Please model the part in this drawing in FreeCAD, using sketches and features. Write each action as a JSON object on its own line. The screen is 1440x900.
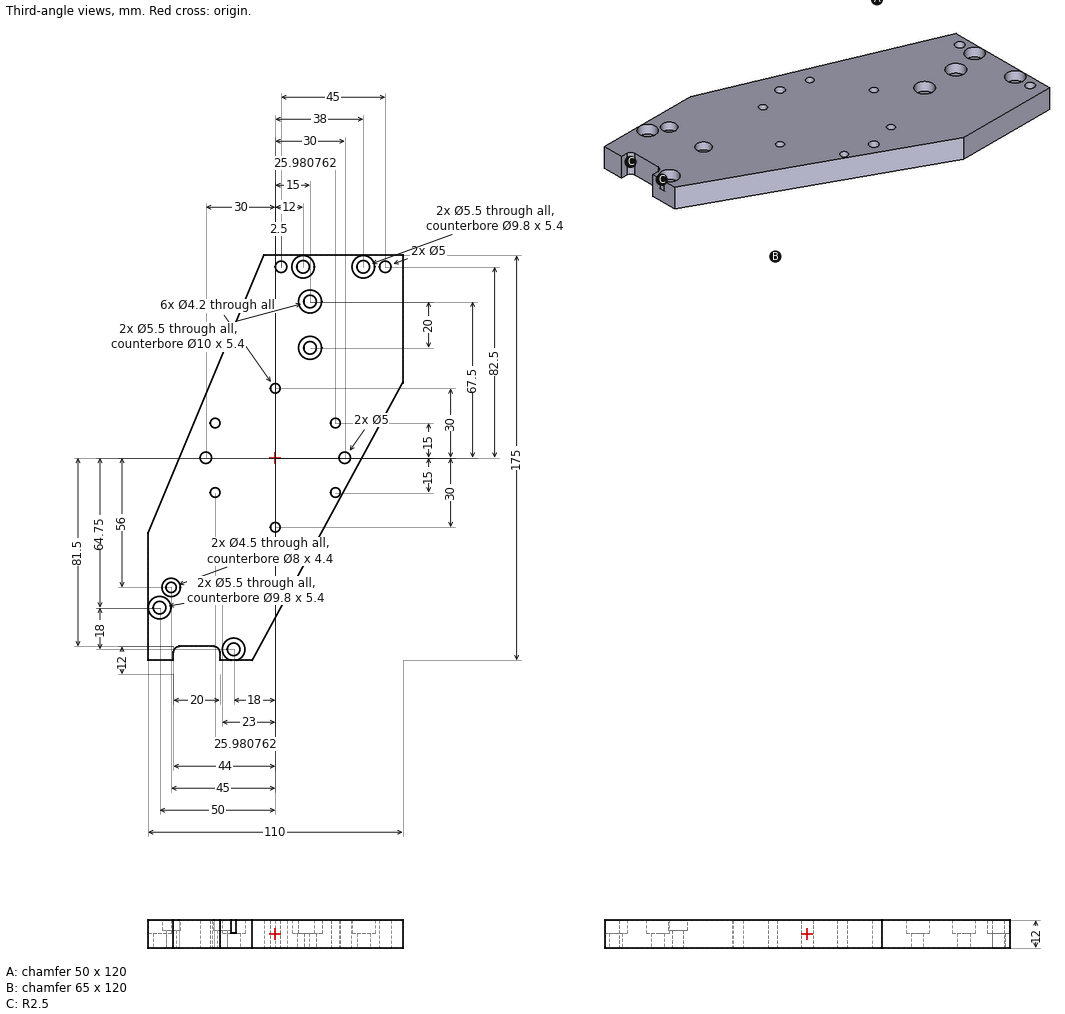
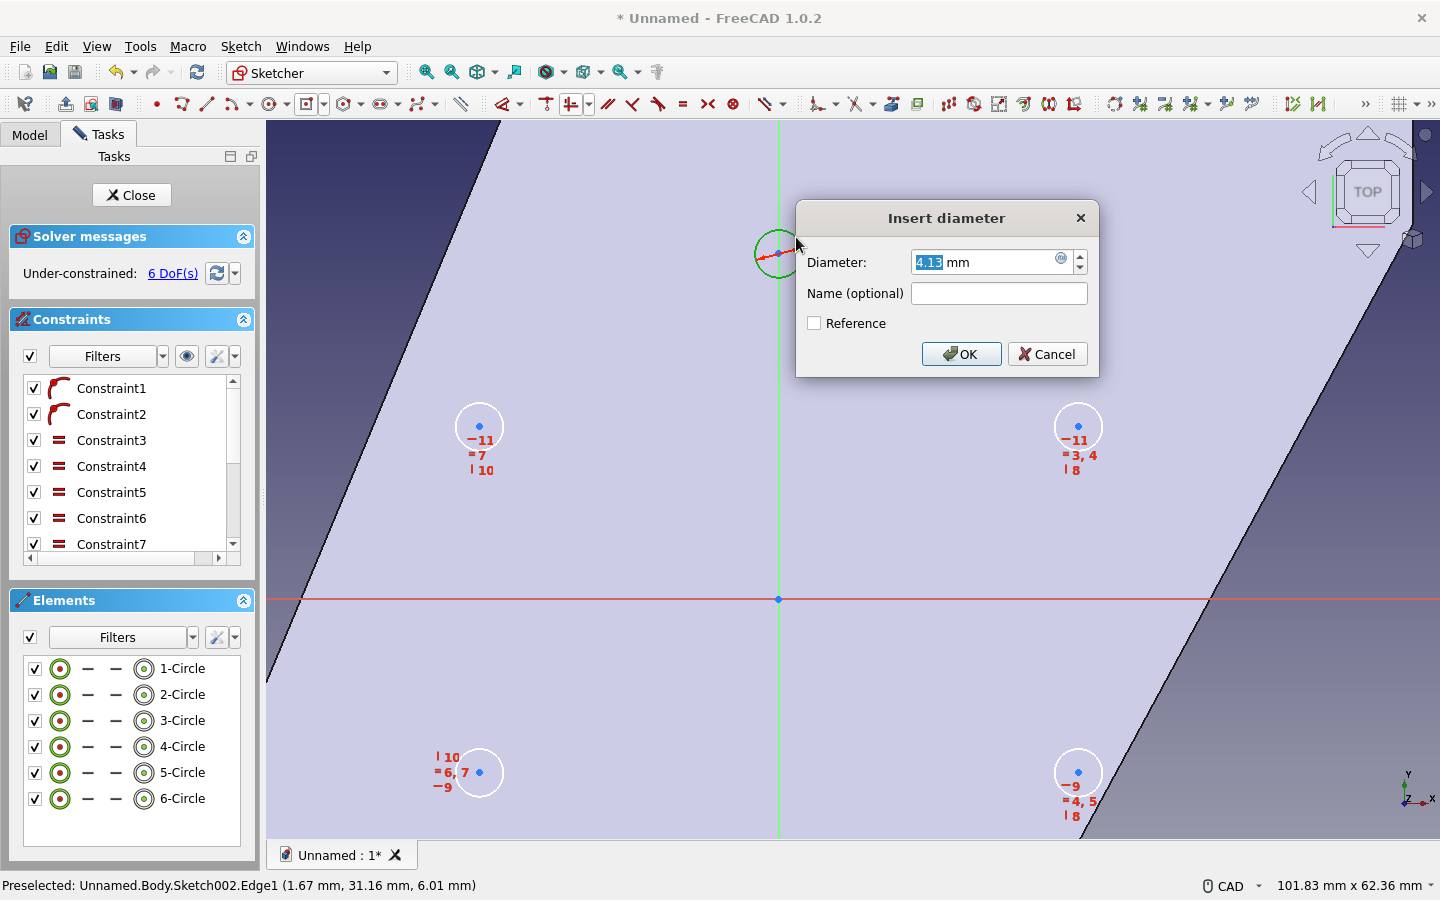
{"action": "type", "text": "4.2"}
{"action": "key", "text": "Return"}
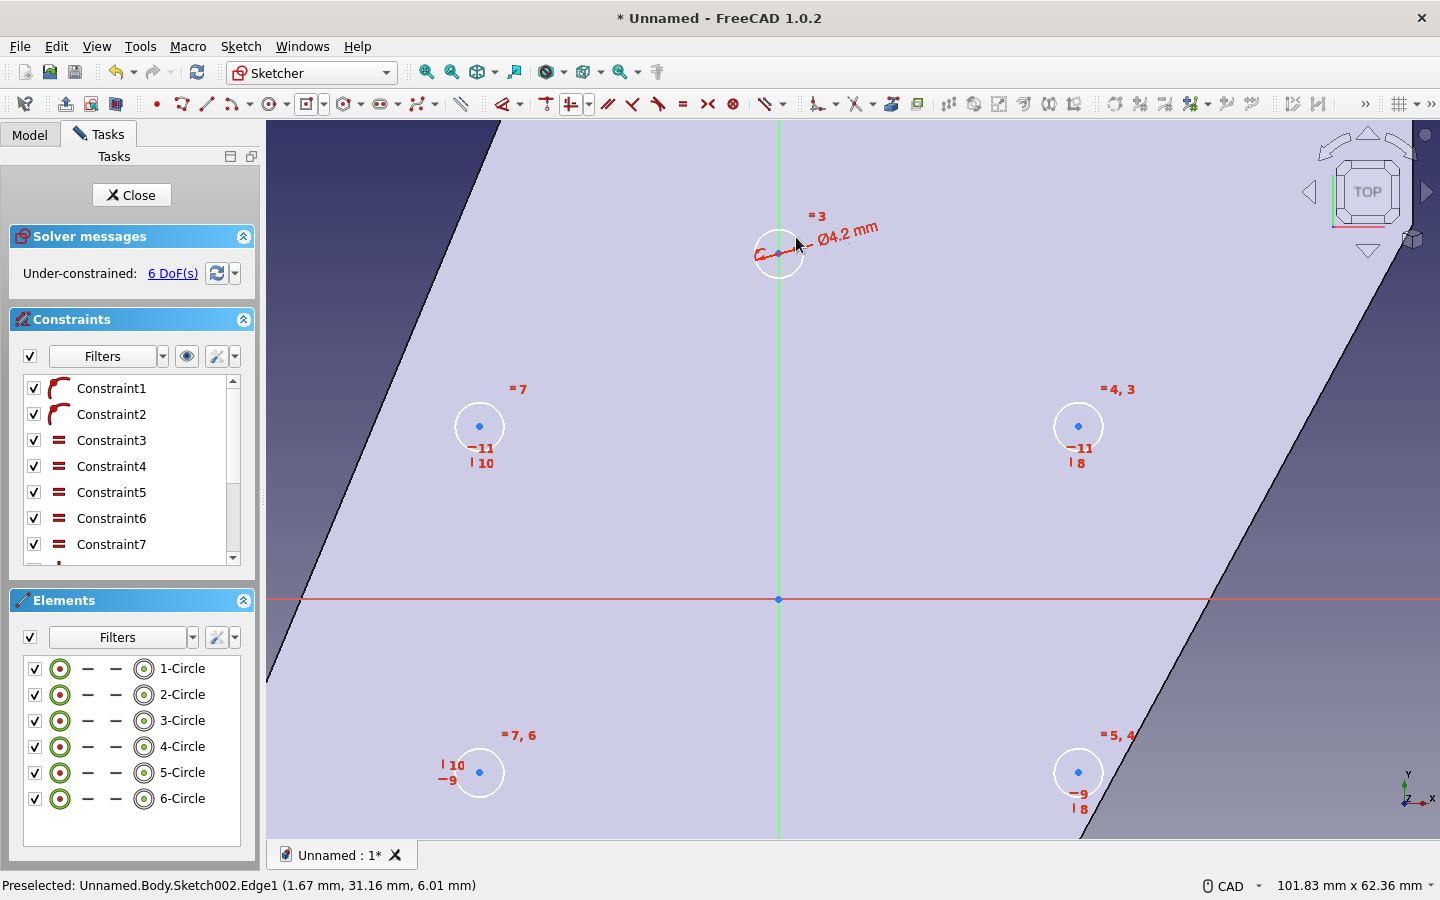
{"action": "left_click", "coordinate": [779, 254]}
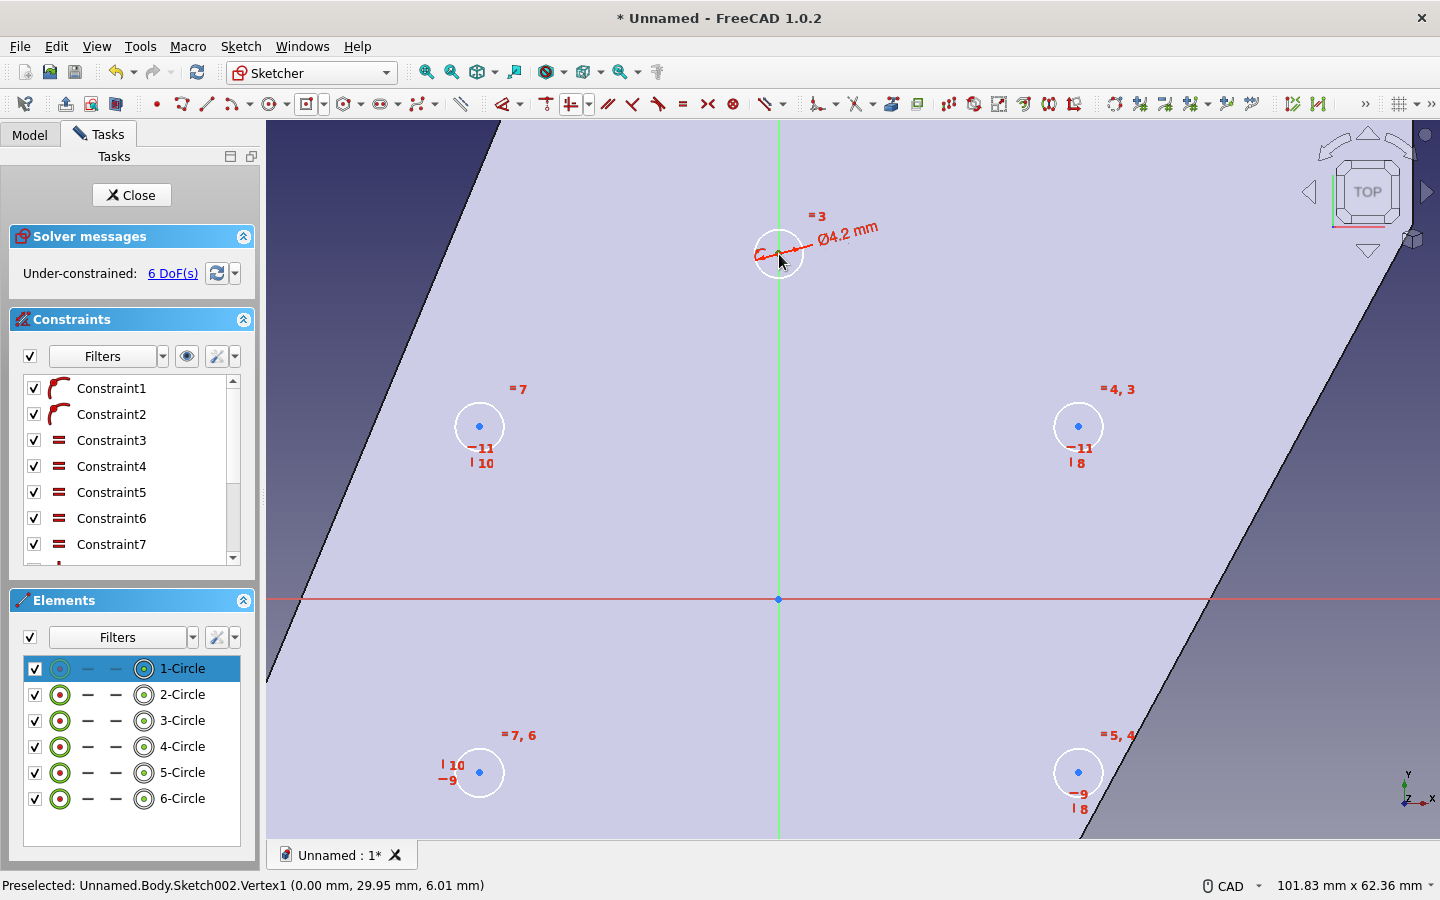
{"action": "key", "text": "i"}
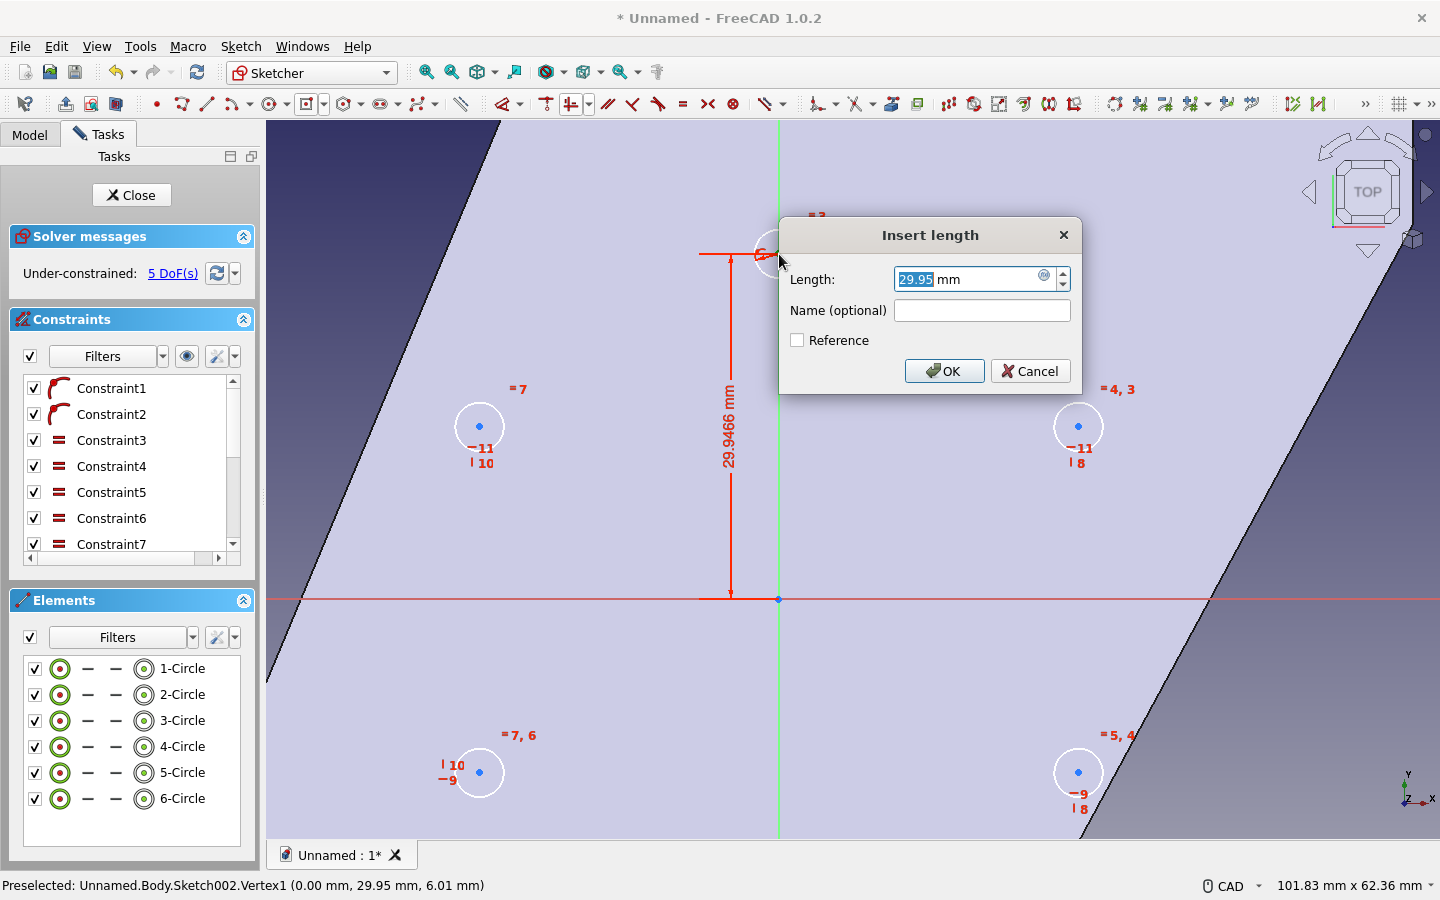
{"action": "type", "text": "30"}
{"action": "key", "text": "Return"}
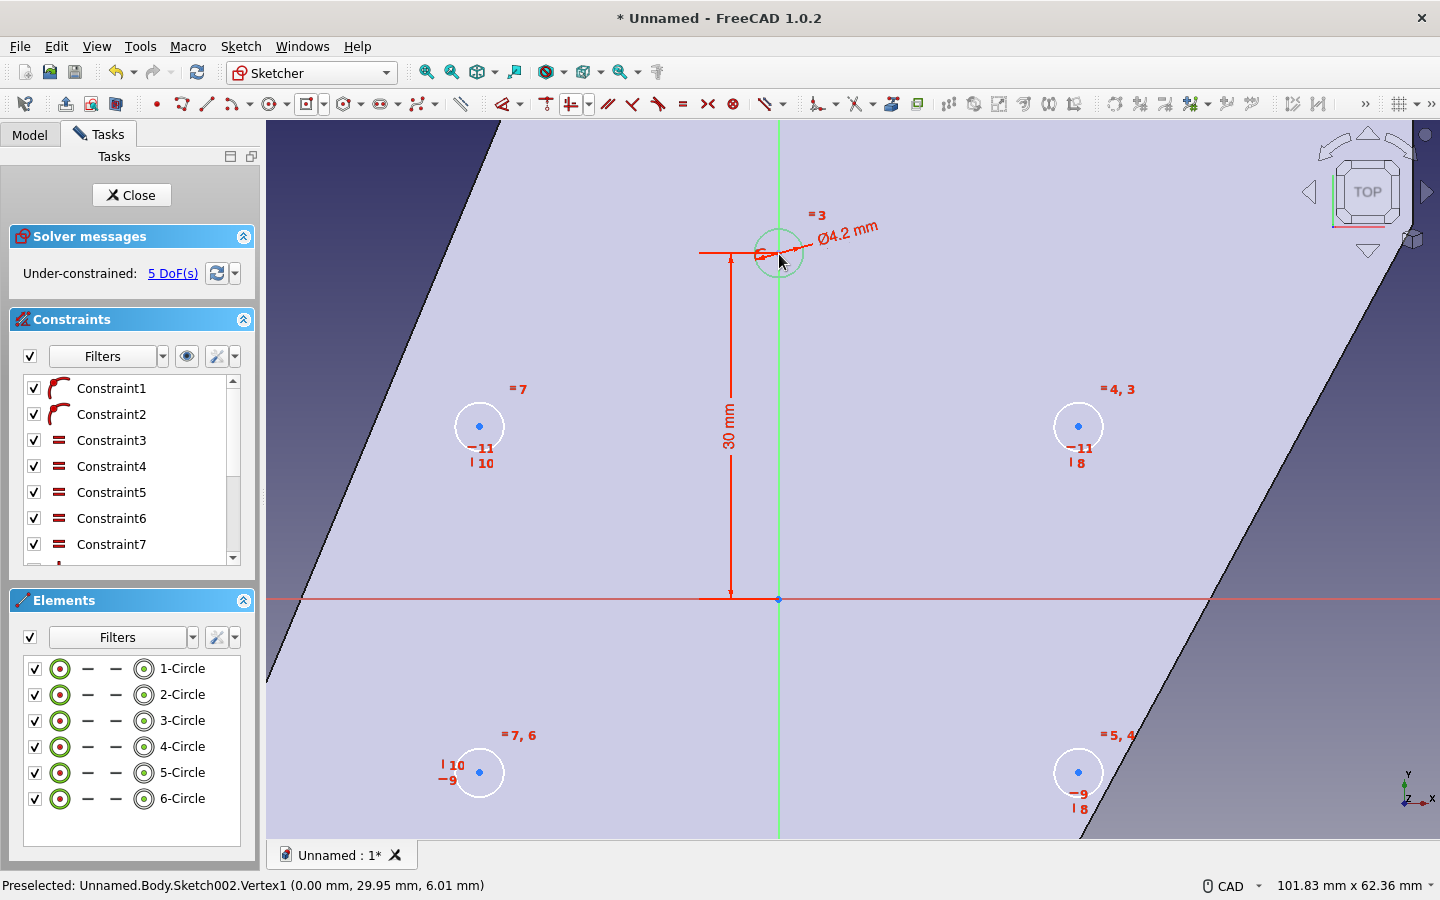
{"action": "left_click", "coordinate": [1079, 427]}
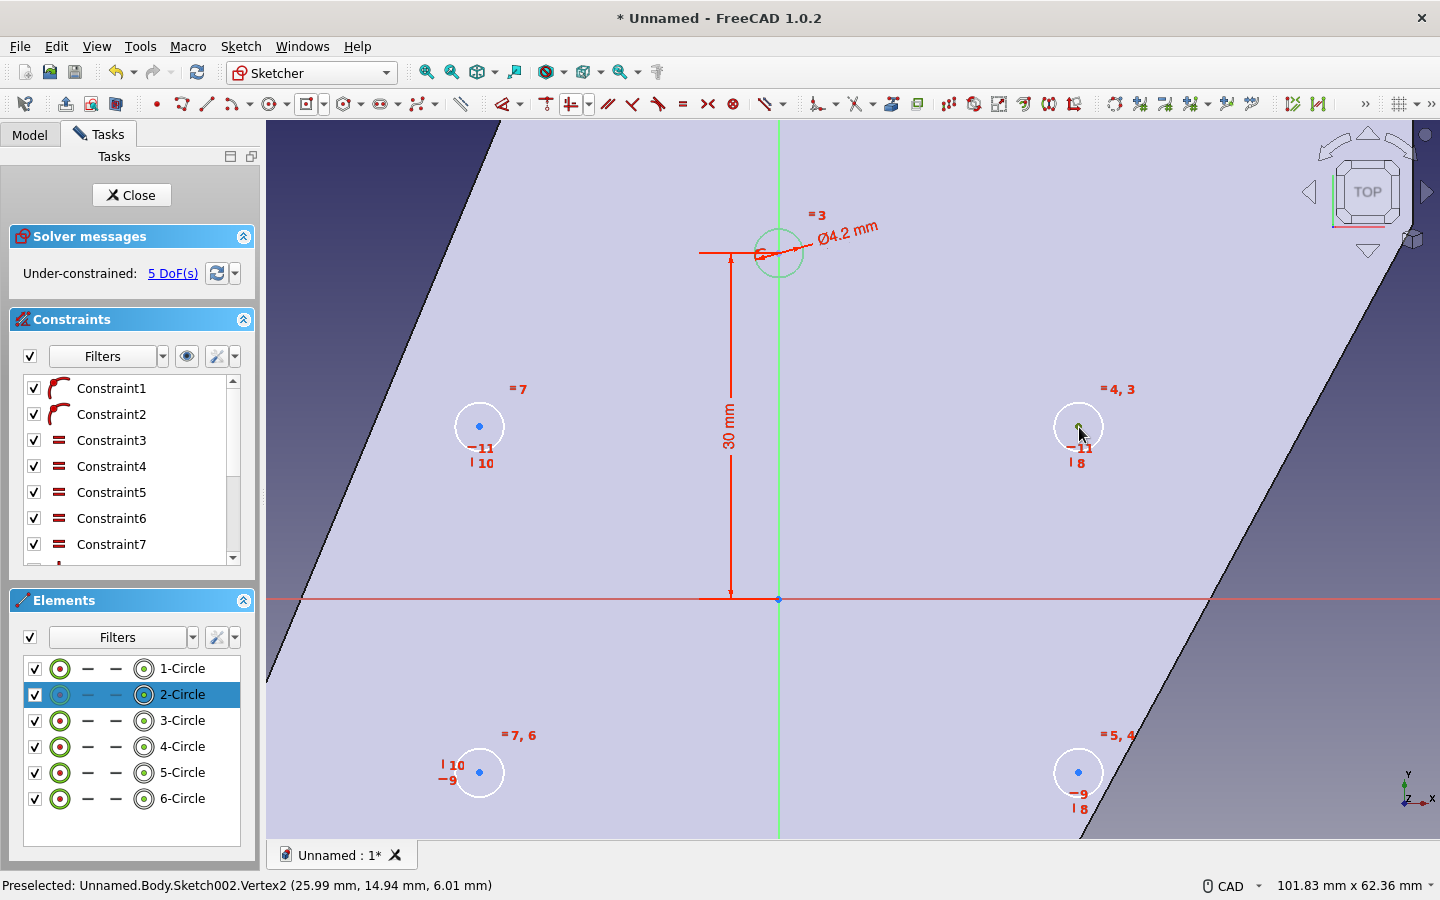
{"action": "key", "text": "i"}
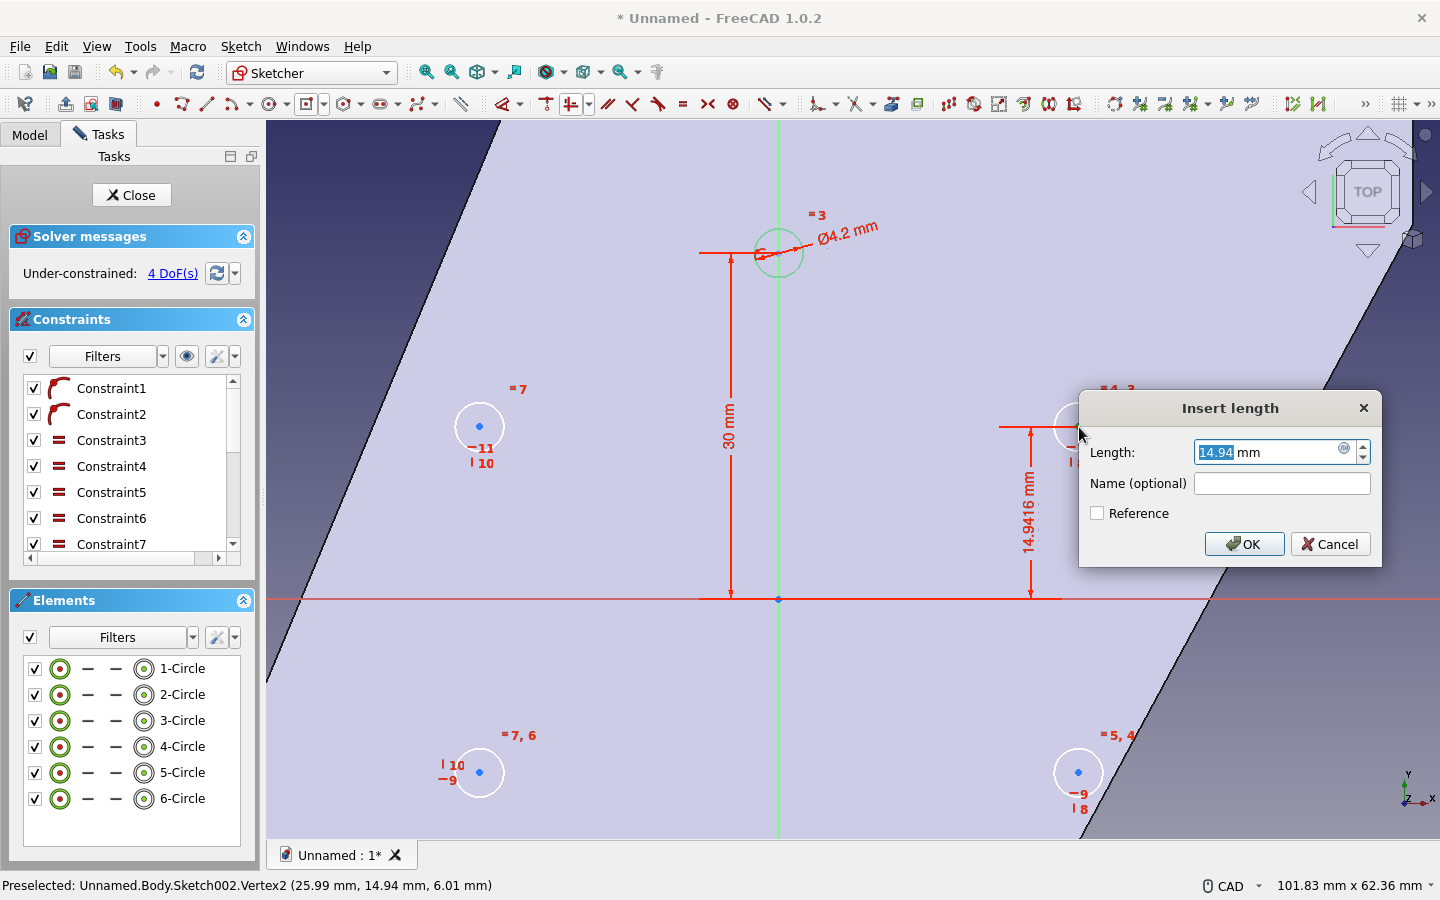
{"action": "type", "text": "15"}
{"action": "key", "text": "Return"}